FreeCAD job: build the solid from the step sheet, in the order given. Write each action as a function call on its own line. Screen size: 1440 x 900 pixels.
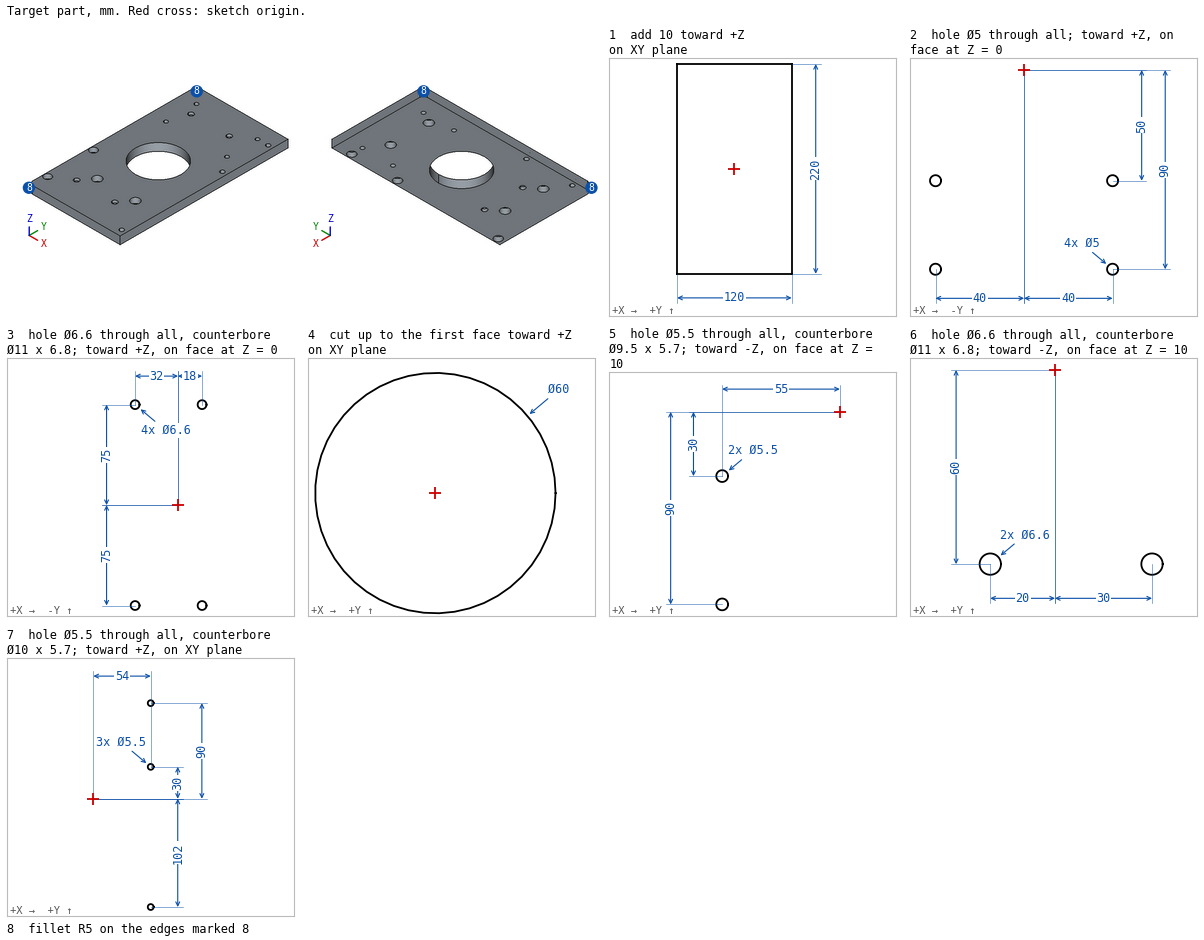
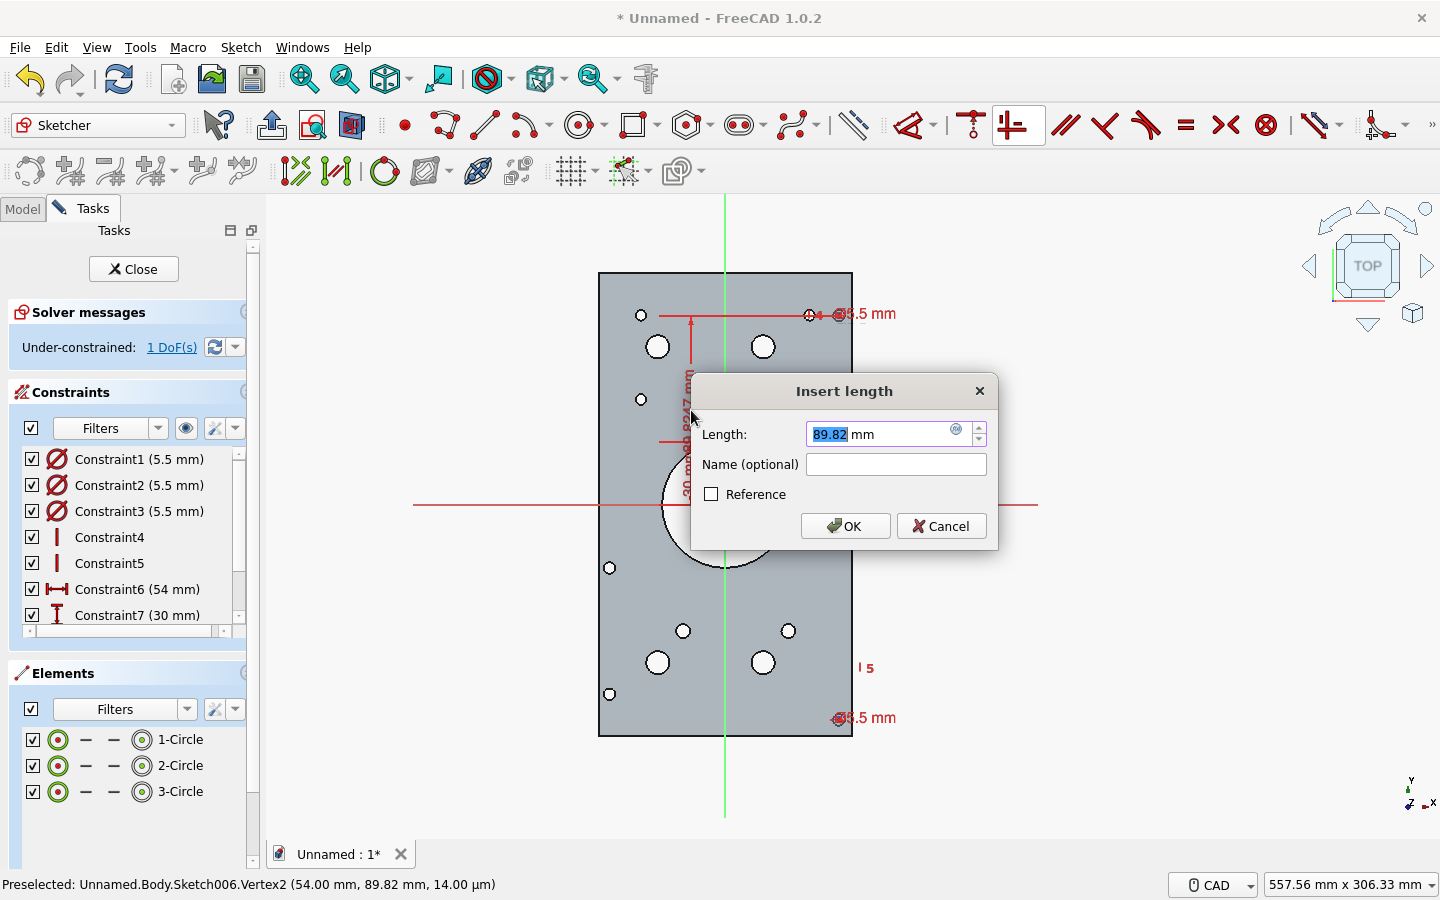
text(90)
key(Return)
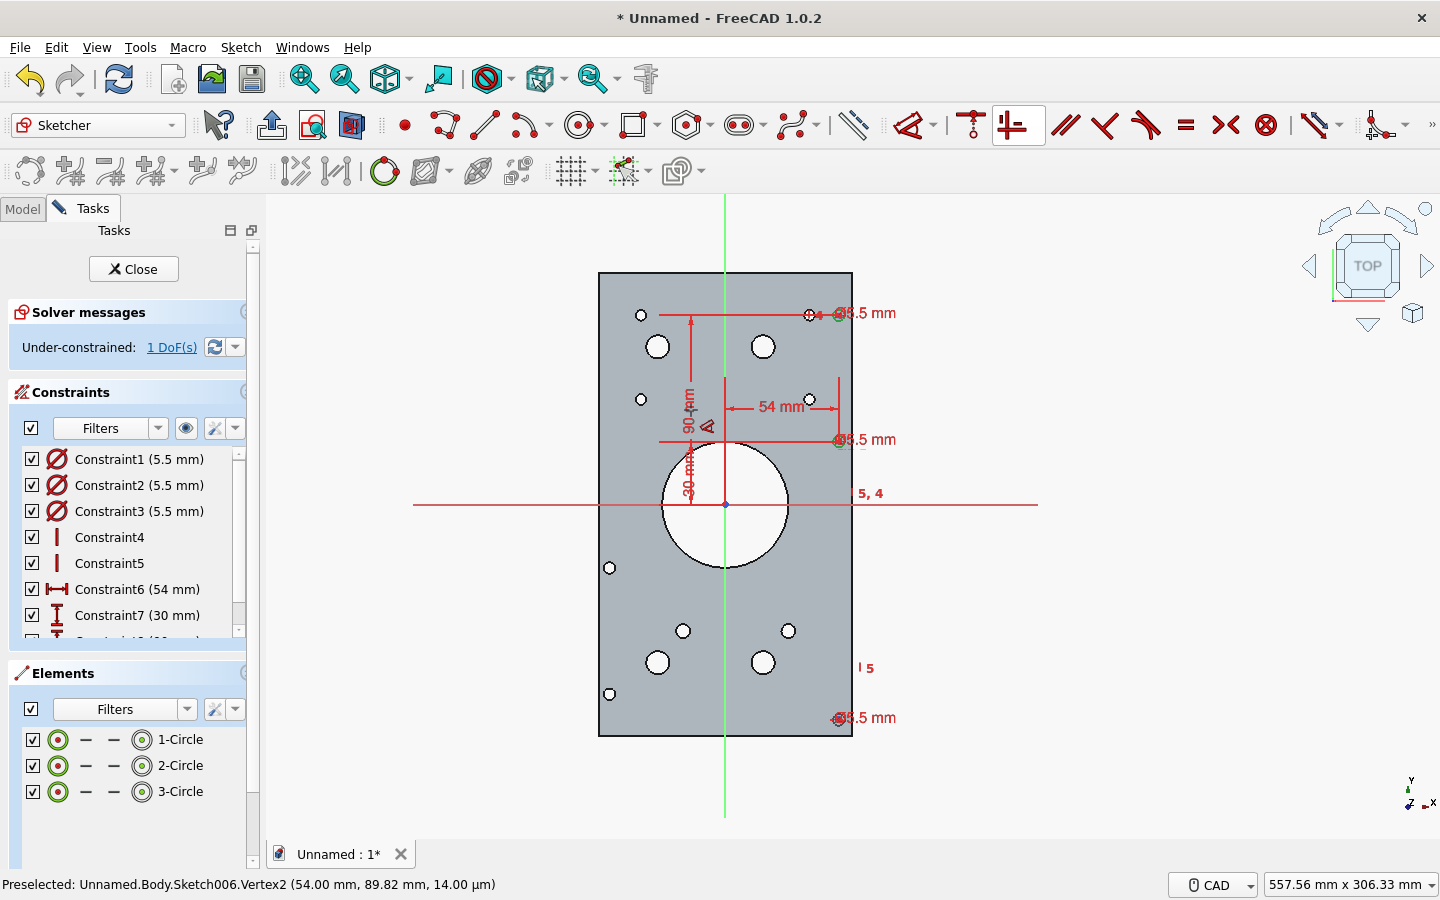
click(839, 720)
click(691, 612)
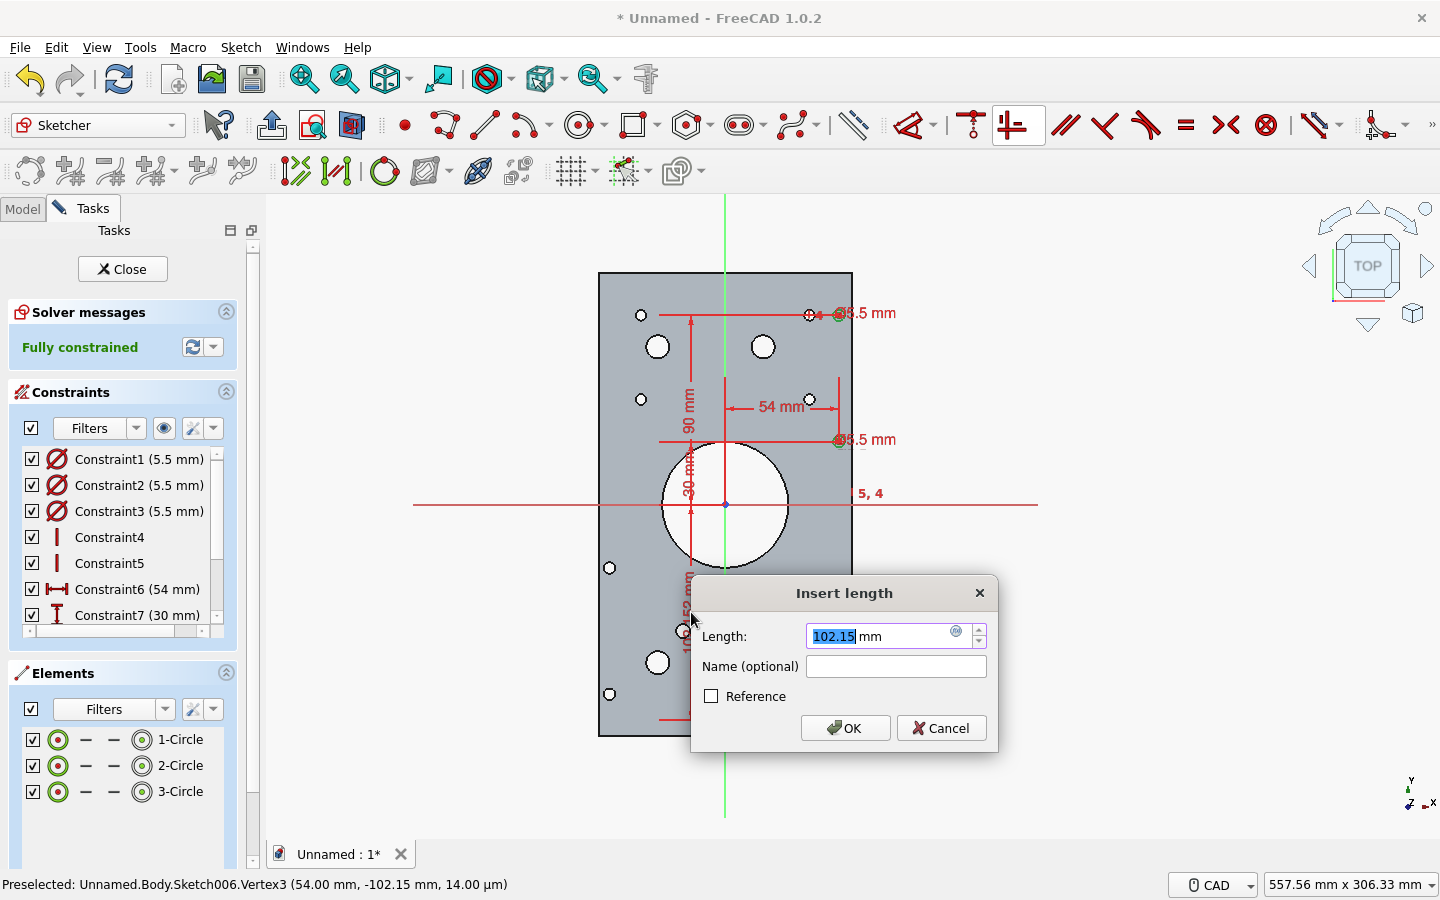
text(102)
key(Return)
key(Escape)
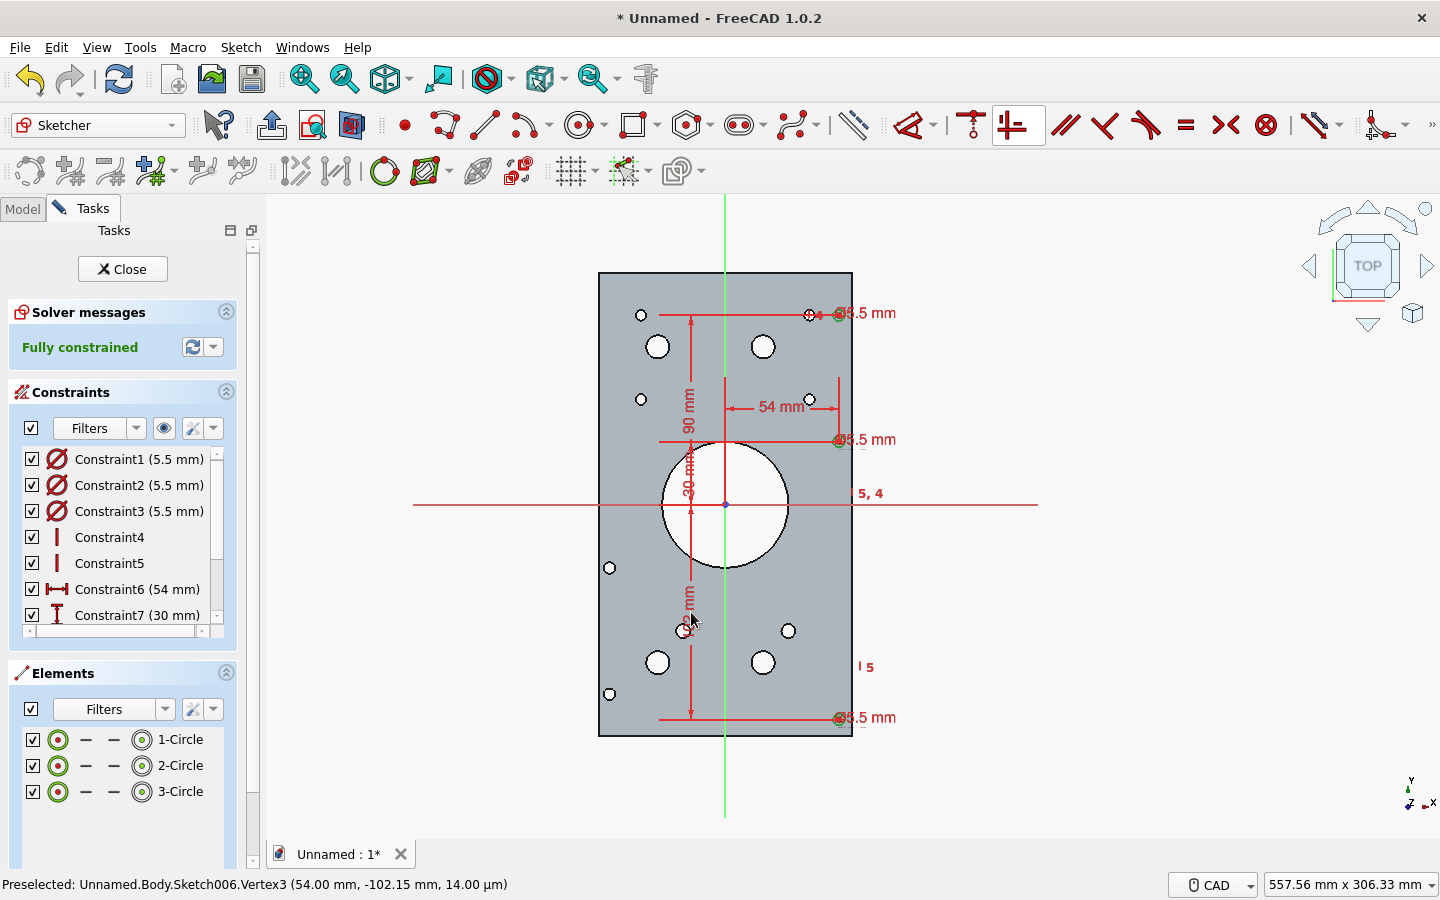
click(123, 269)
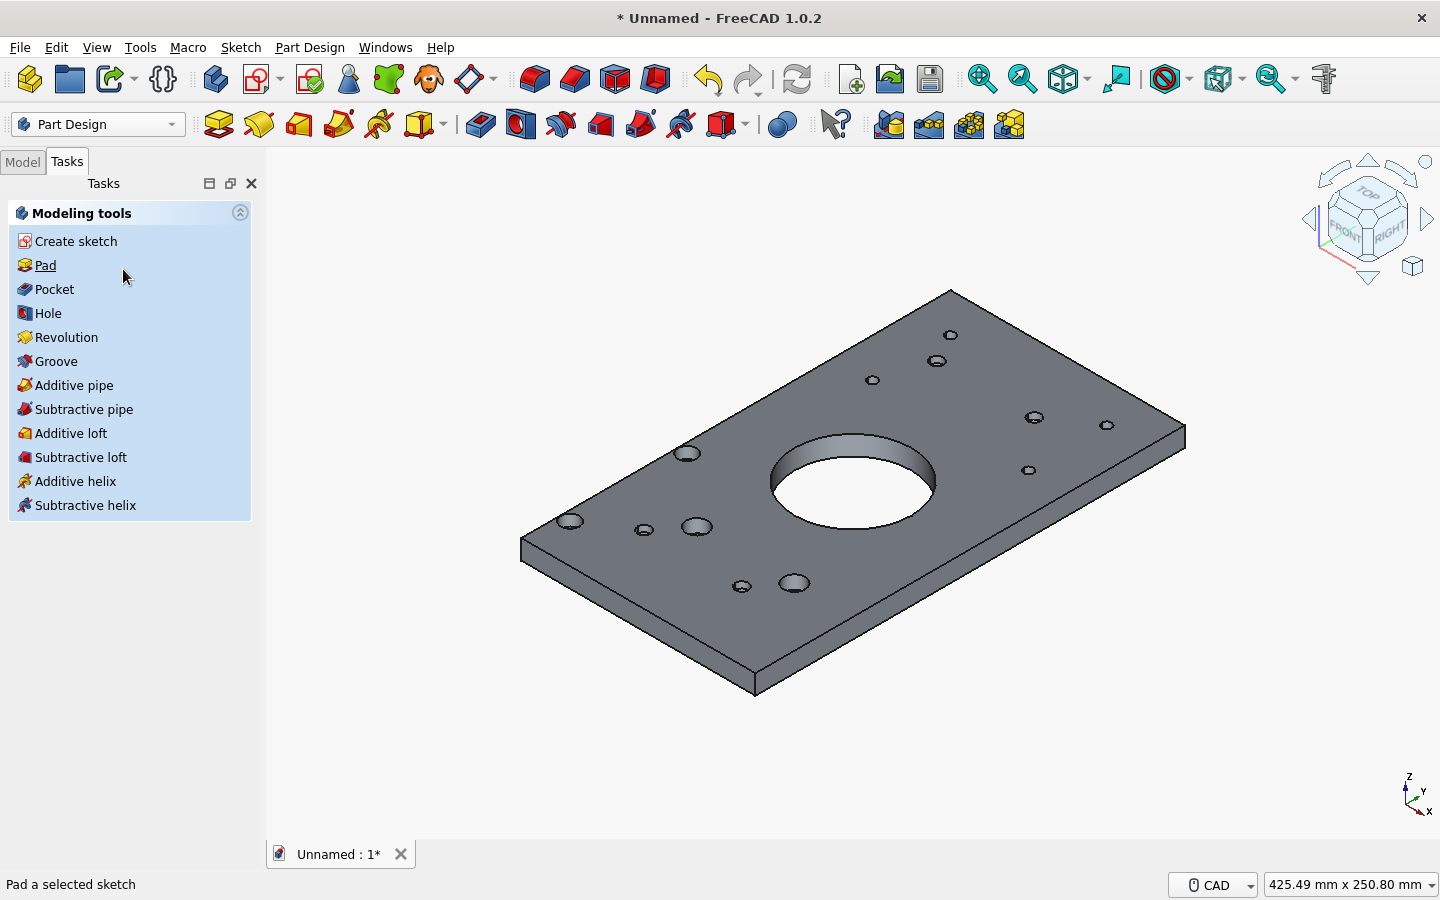
click(522, 124)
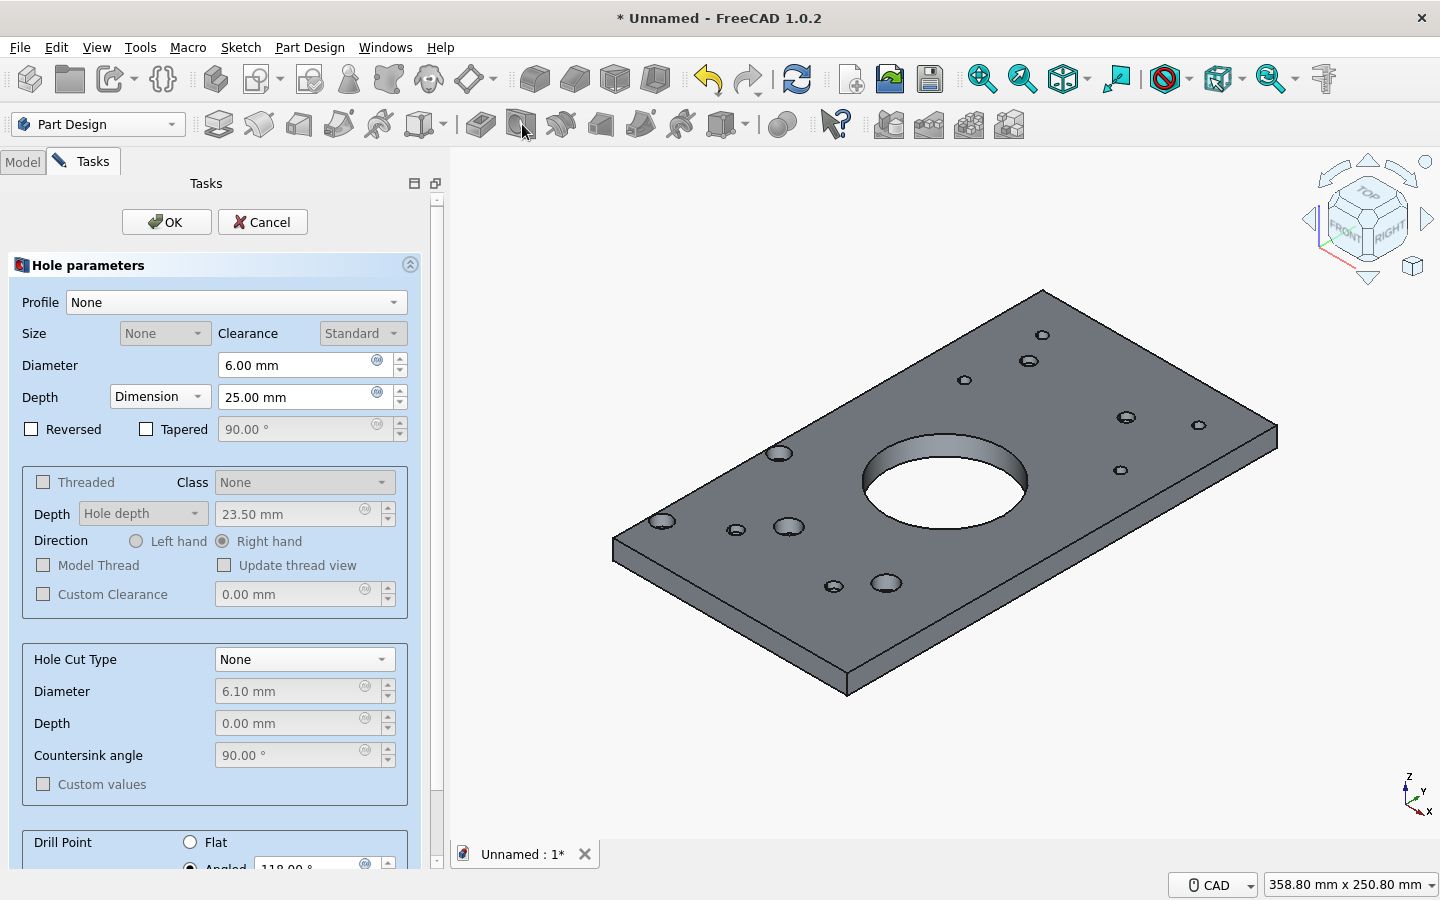
triple_click(305, 365)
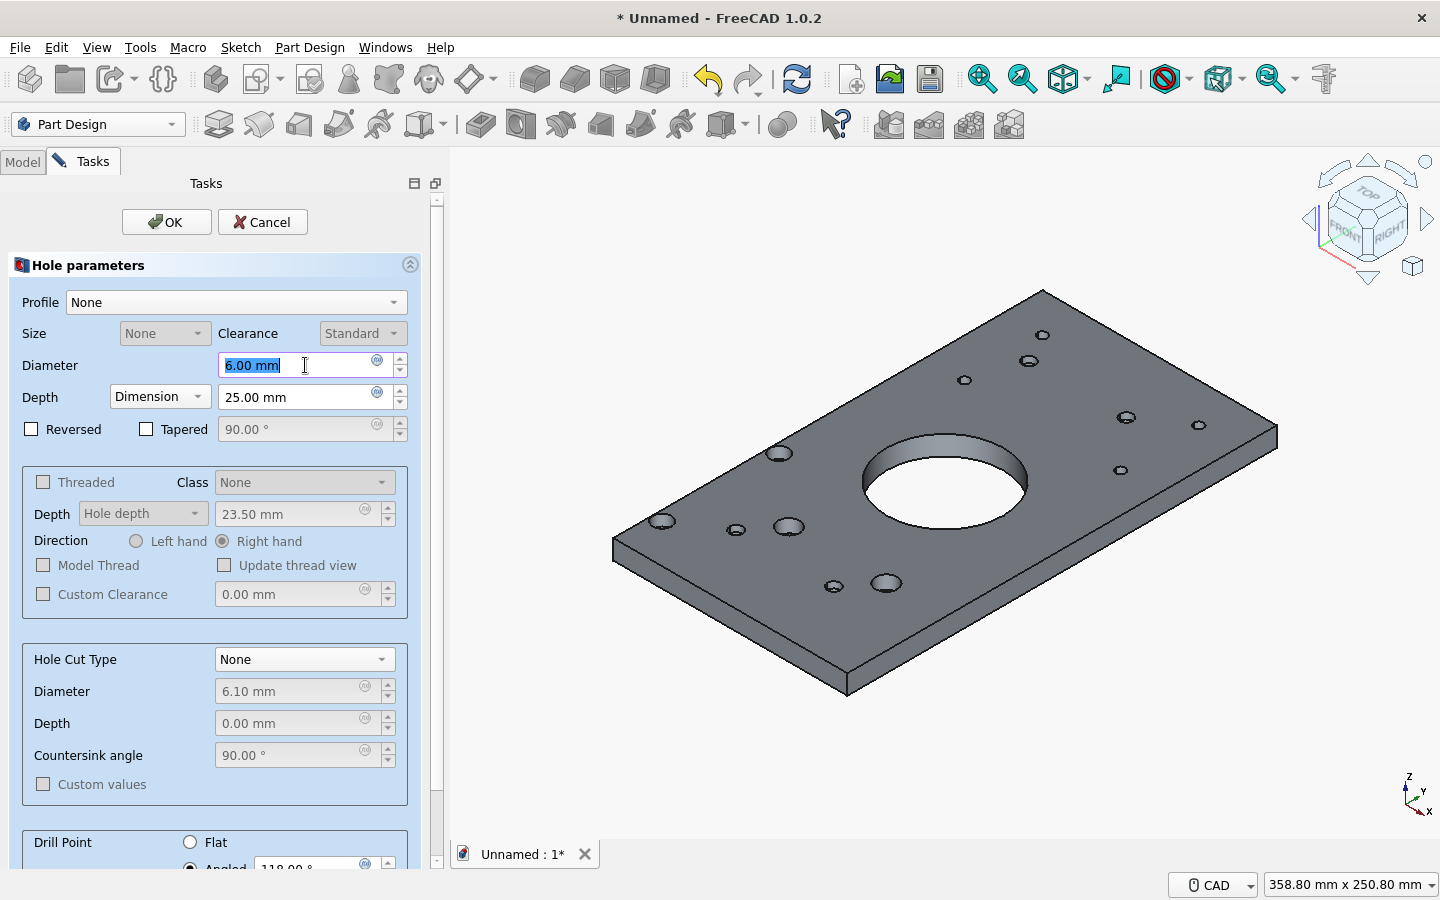
text(5.5)
key(Tab)